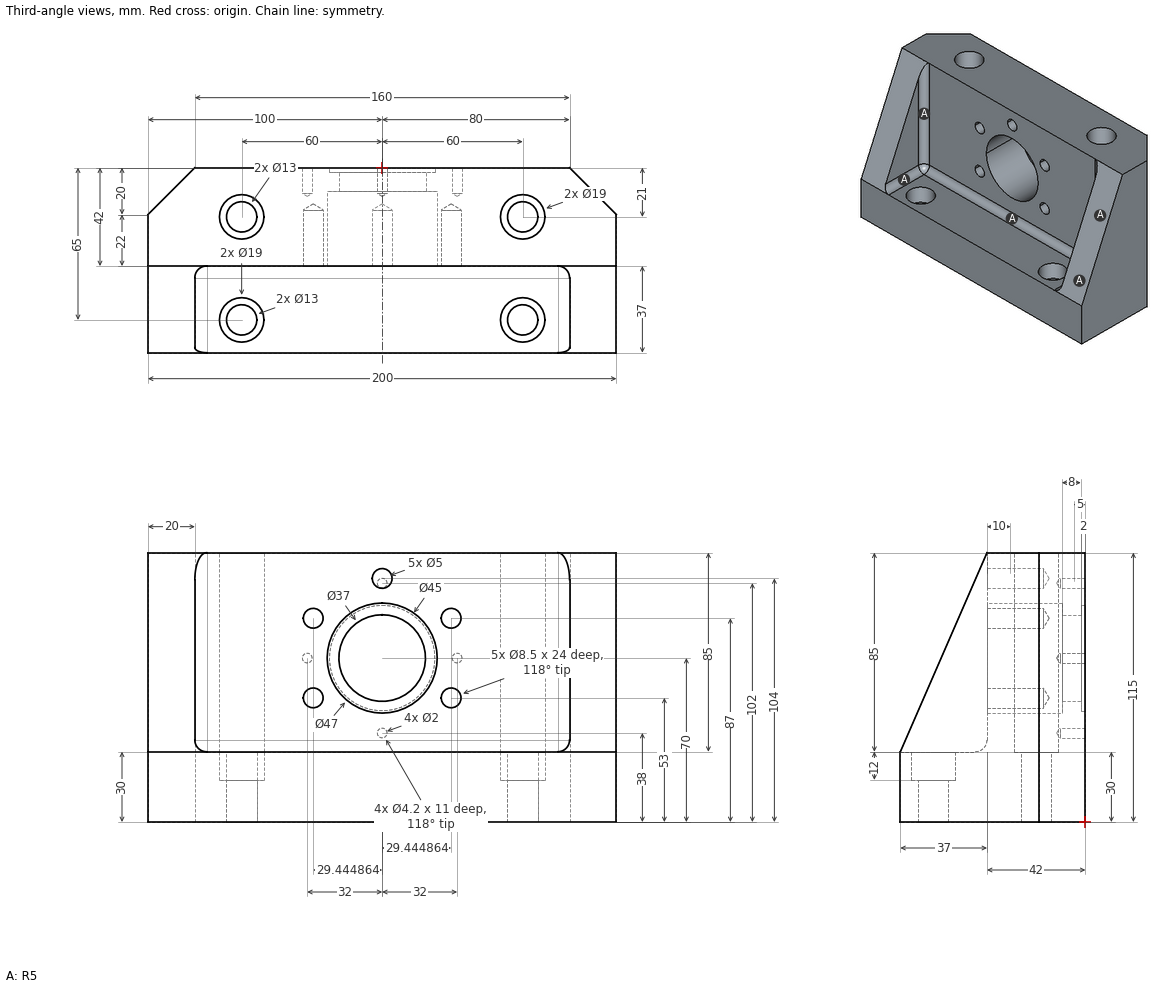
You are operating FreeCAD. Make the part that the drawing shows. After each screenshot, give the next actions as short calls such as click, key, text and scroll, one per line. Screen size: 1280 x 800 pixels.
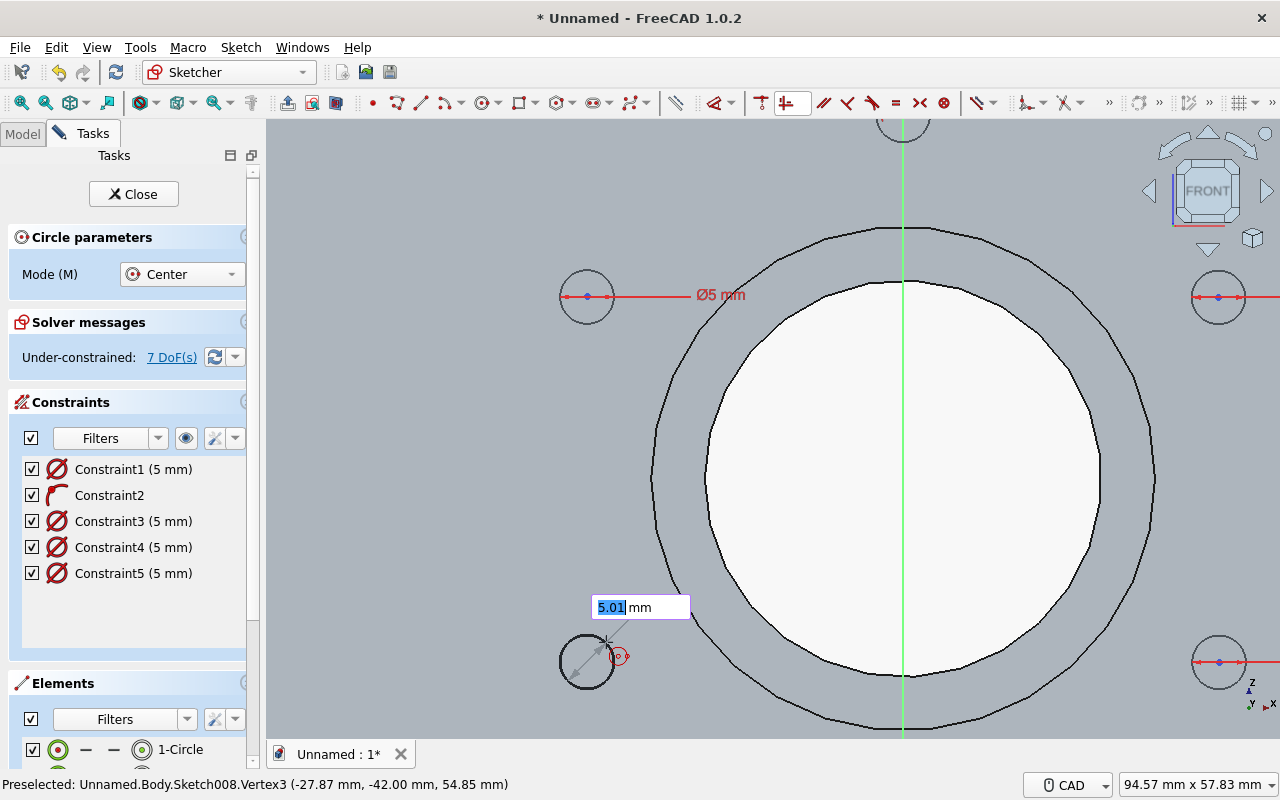
text(5)
key(Return)
key(Escape)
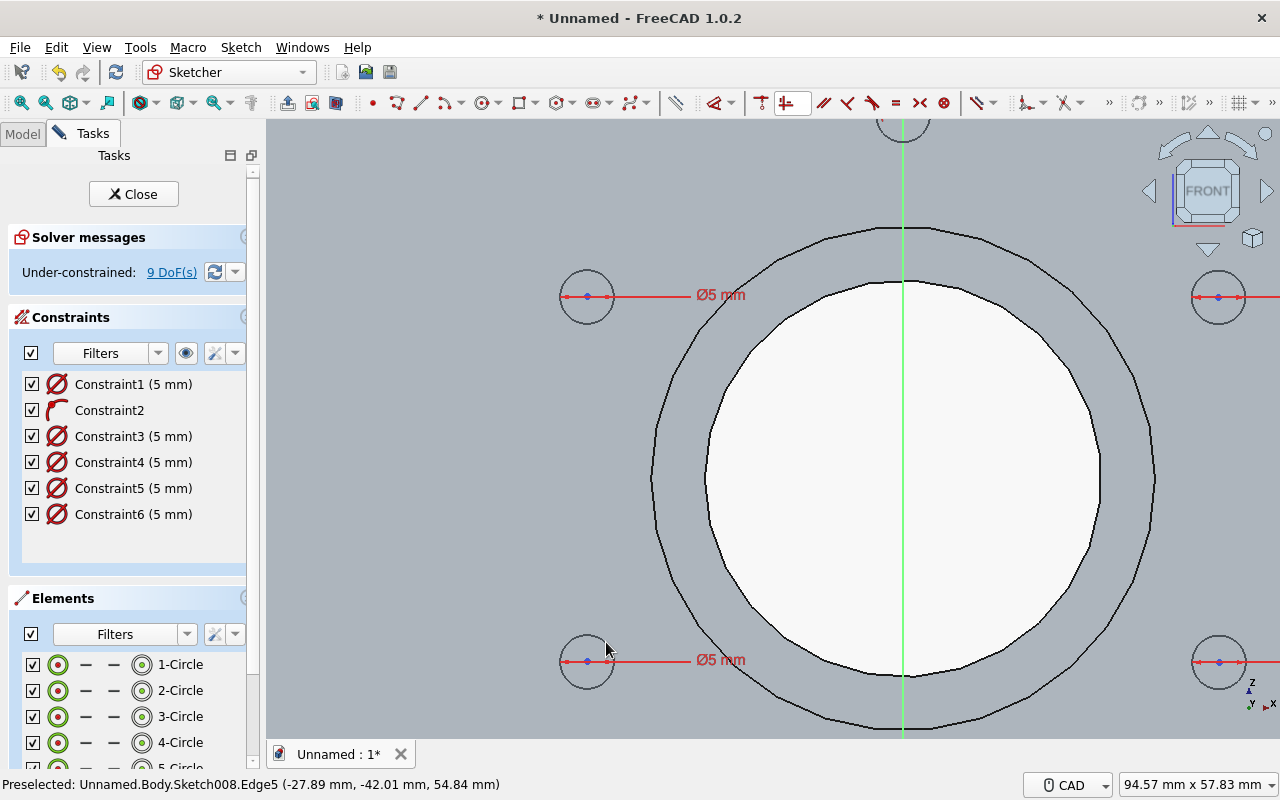
scroll(589, 296, down, 5)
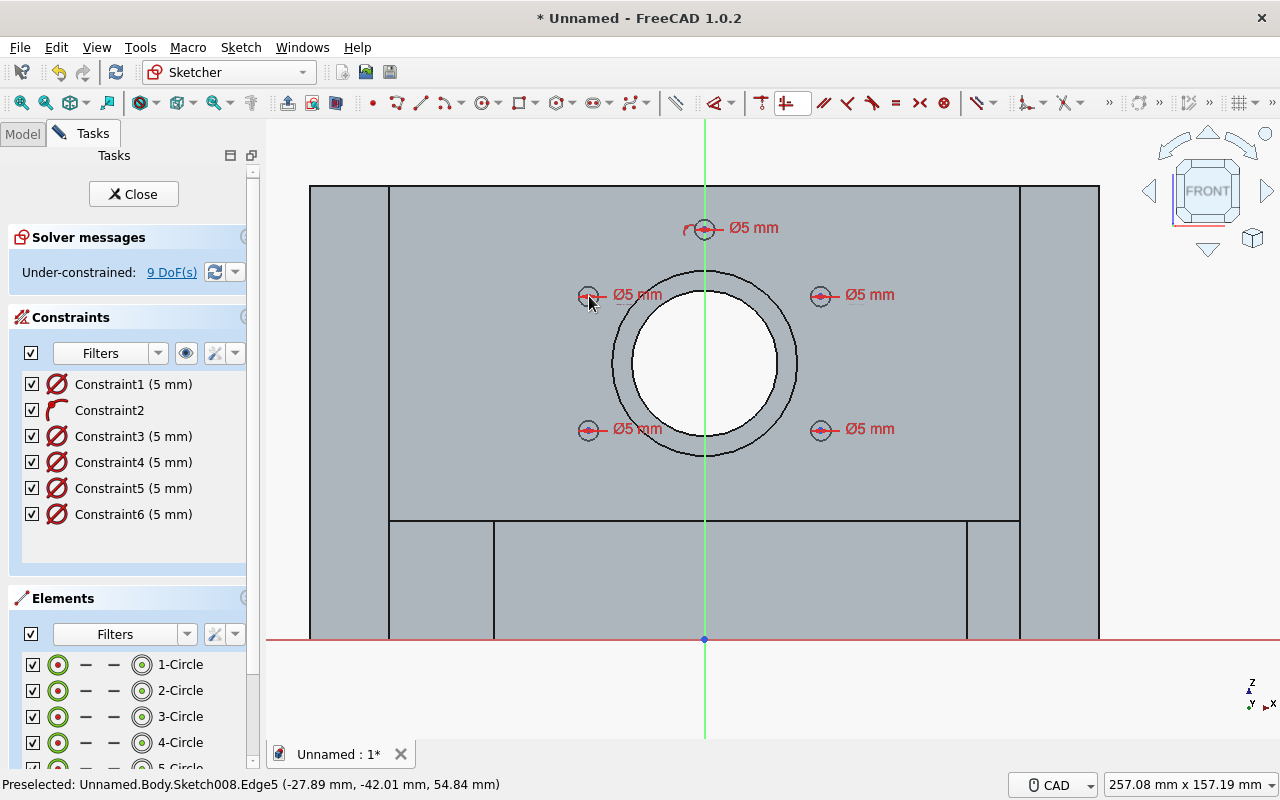
click(821, 297)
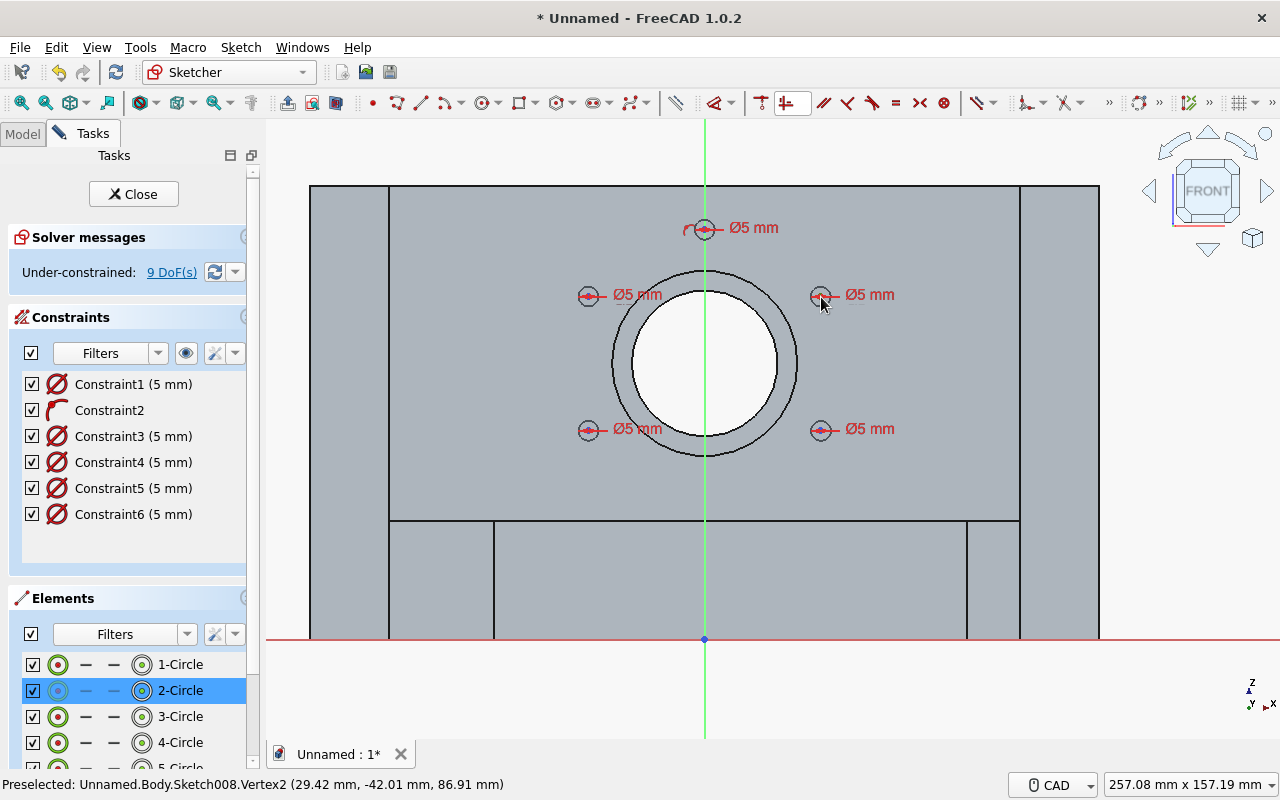
click(821, 431)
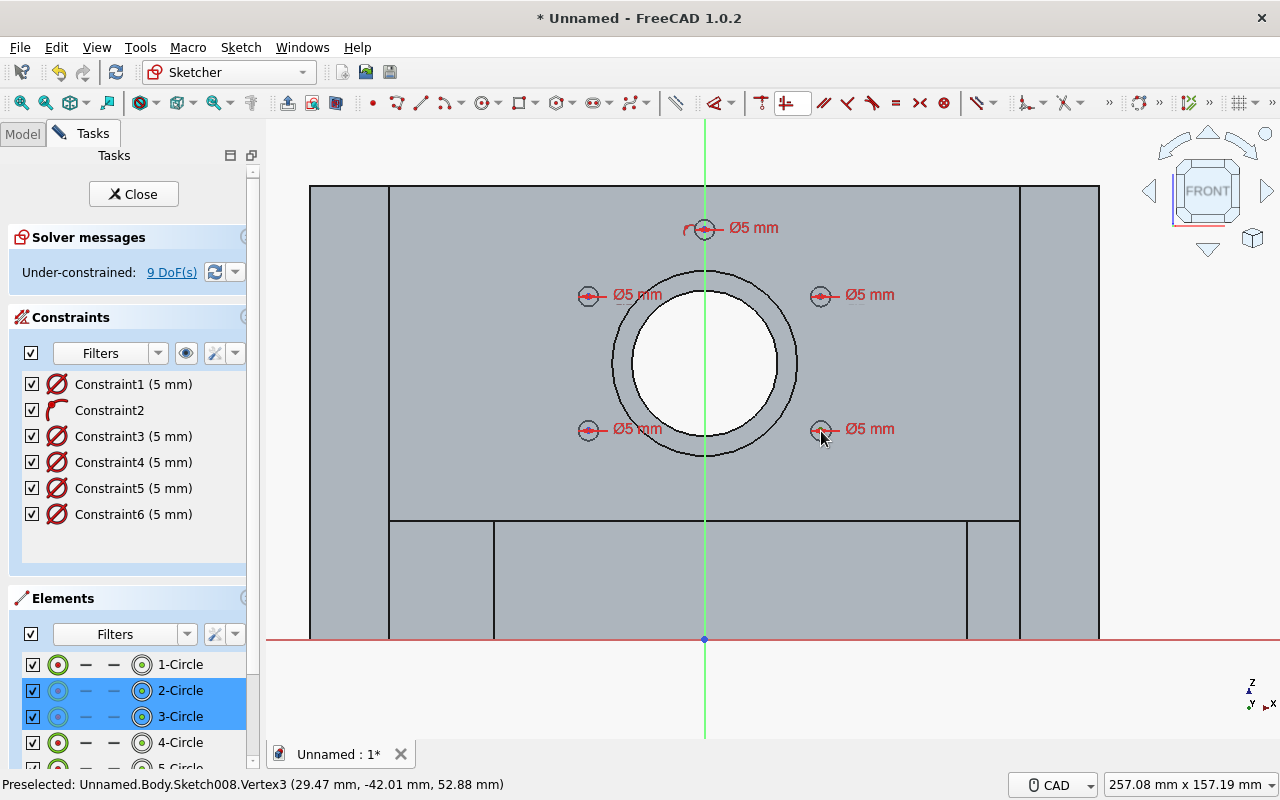
click(806, 104)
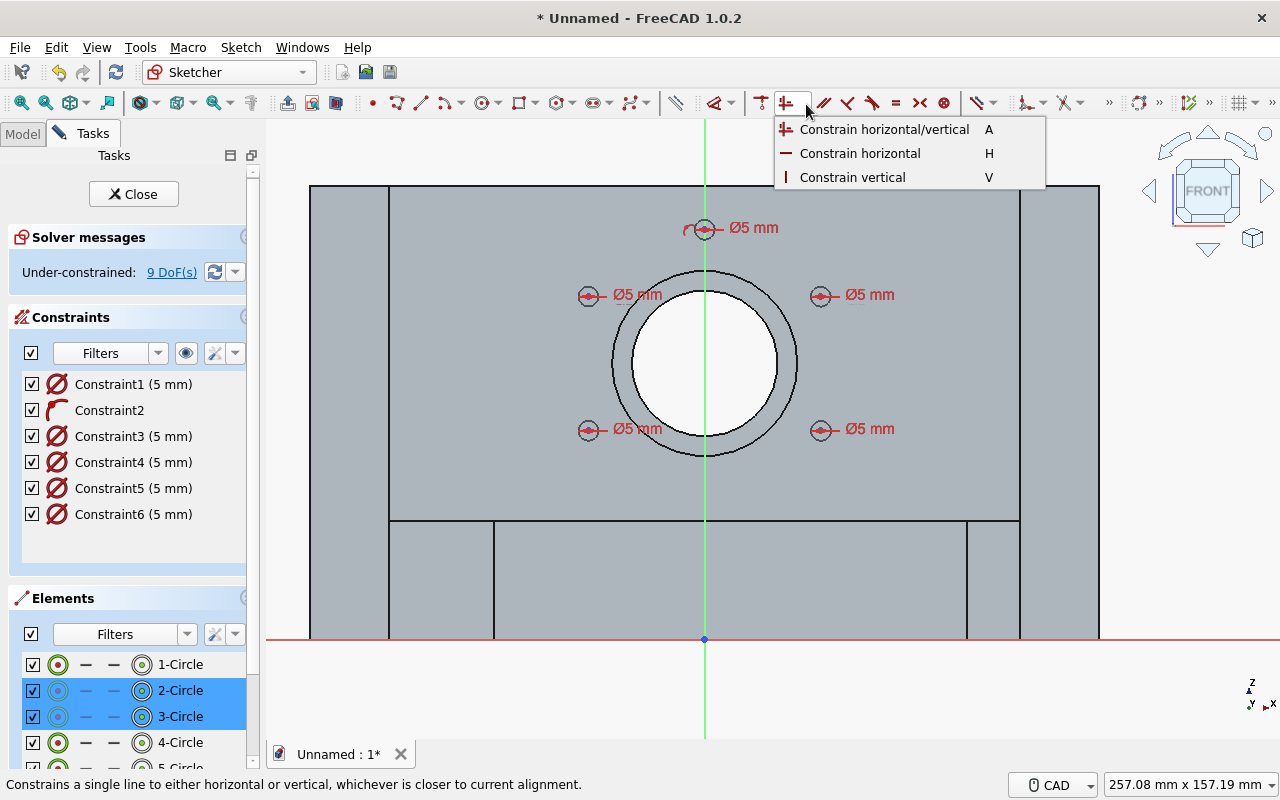
click(910, 177)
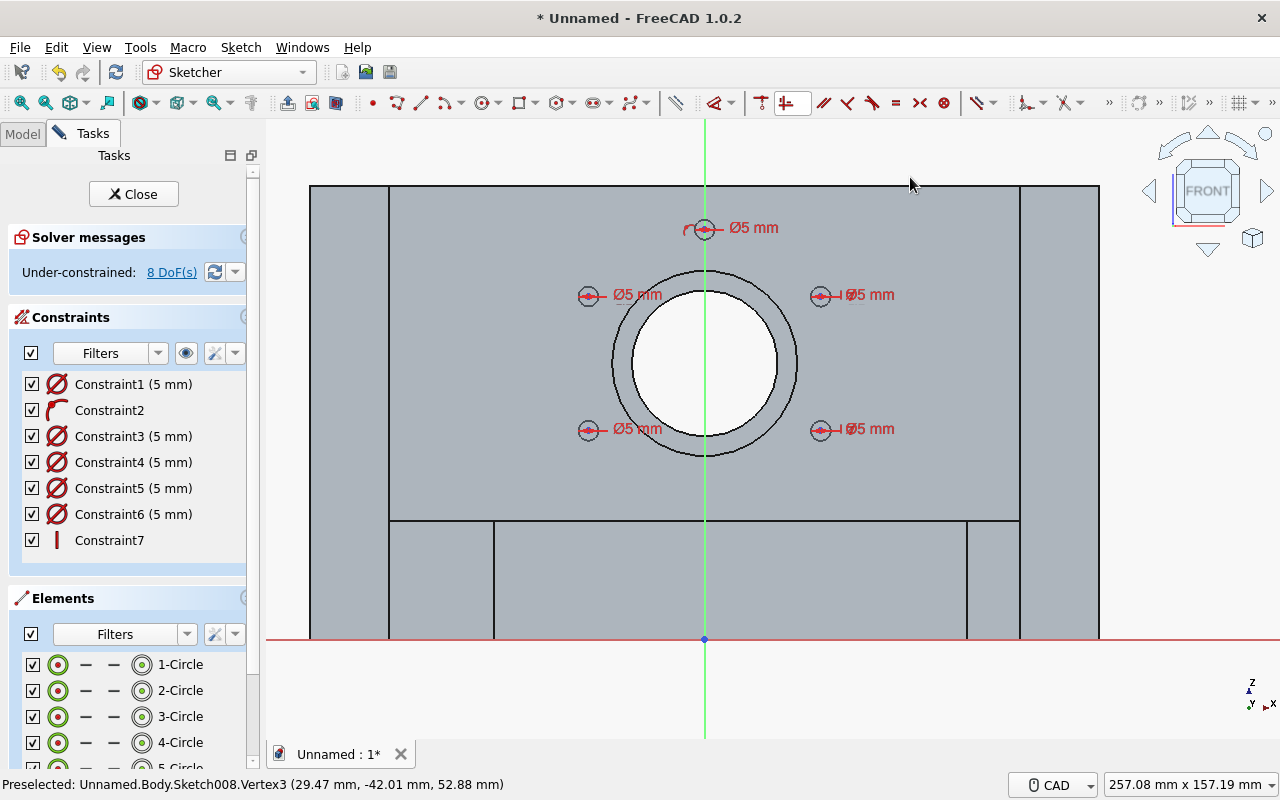
click(821, 297)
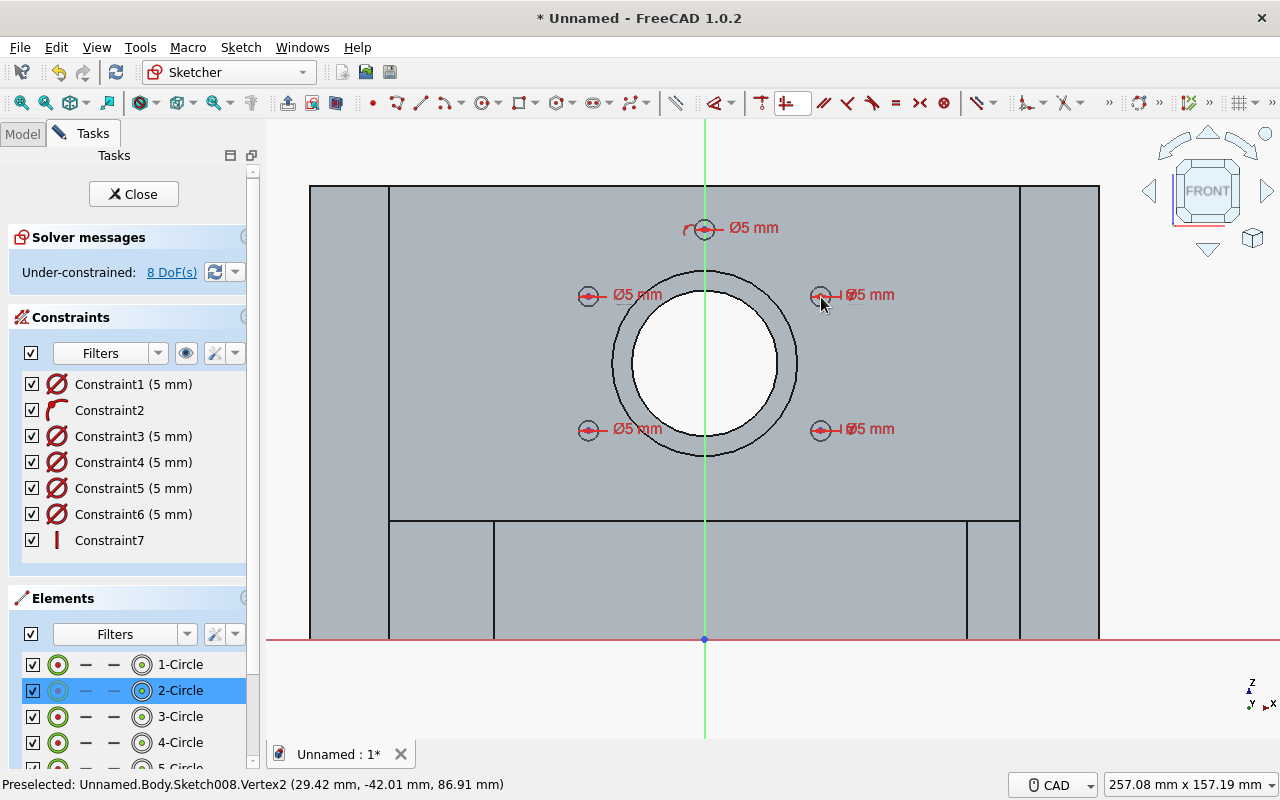
click(588, 297)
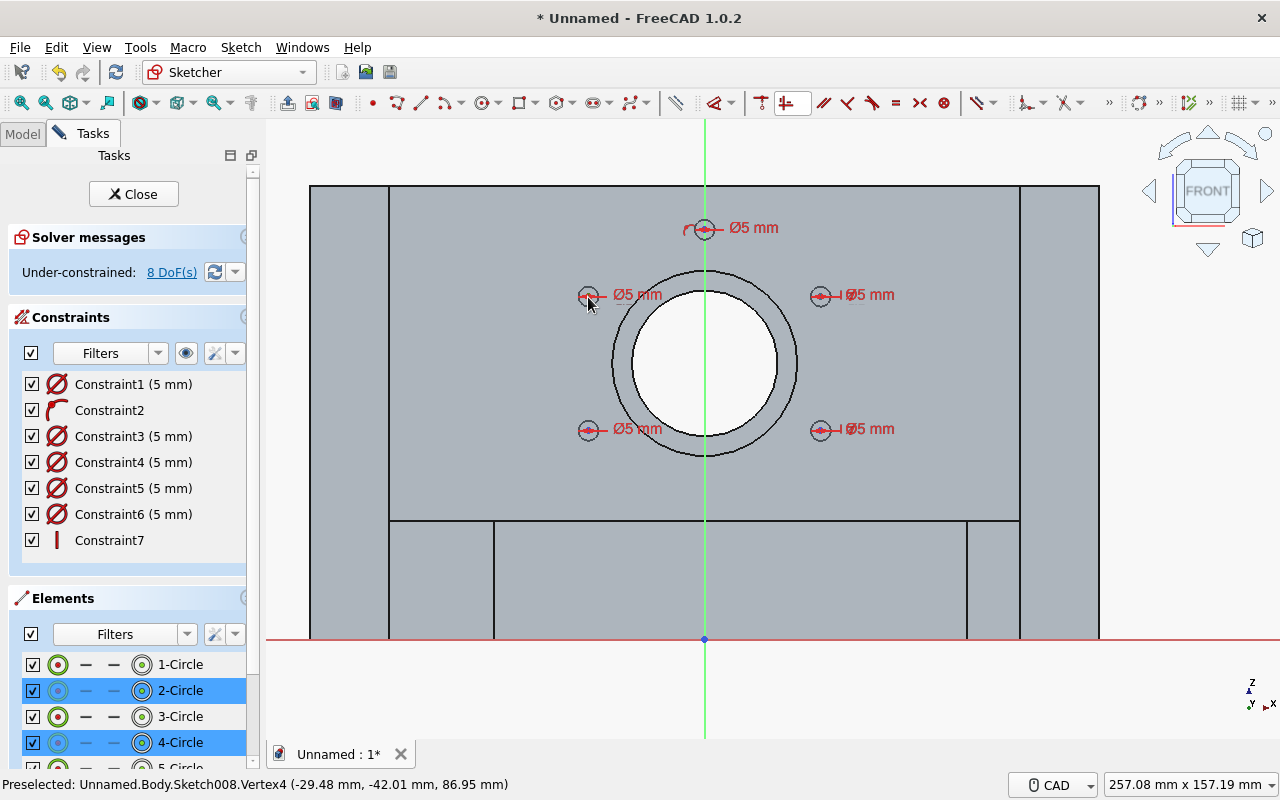
key(h)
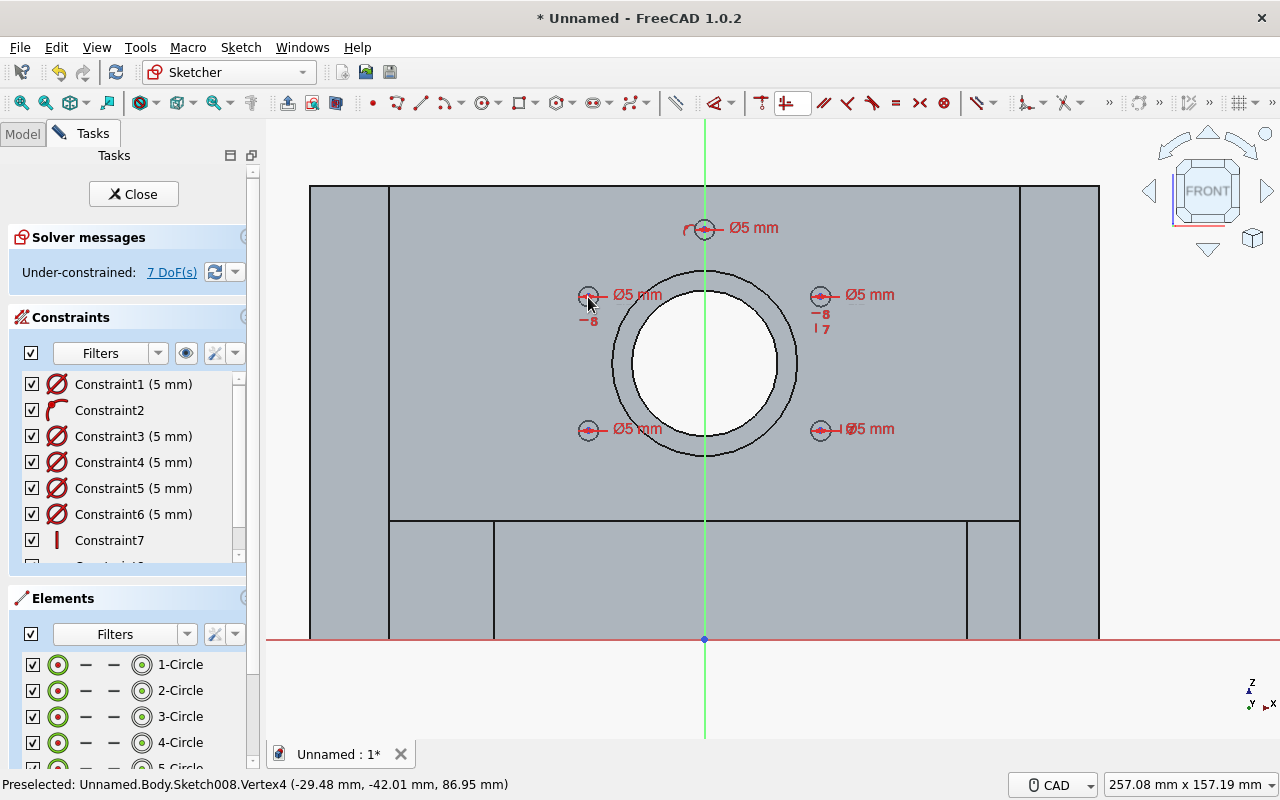
click(588, 297)